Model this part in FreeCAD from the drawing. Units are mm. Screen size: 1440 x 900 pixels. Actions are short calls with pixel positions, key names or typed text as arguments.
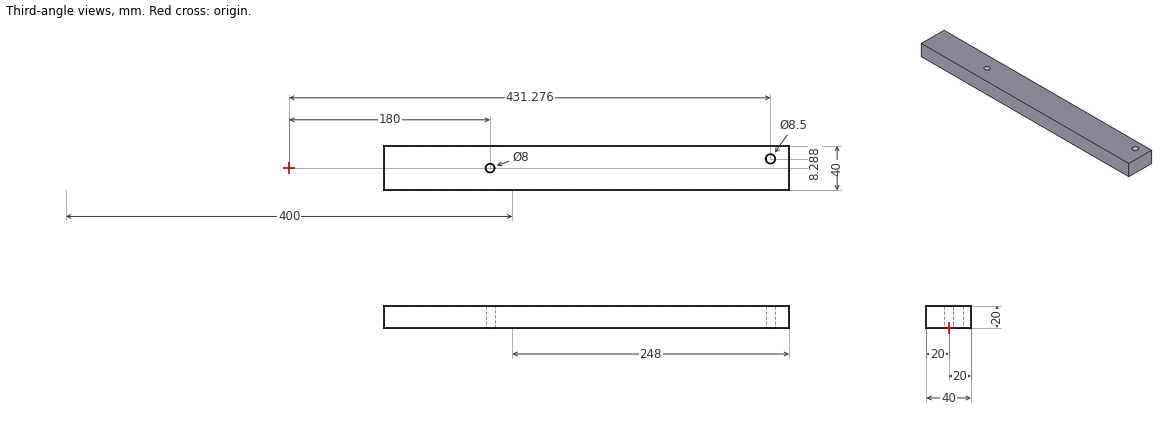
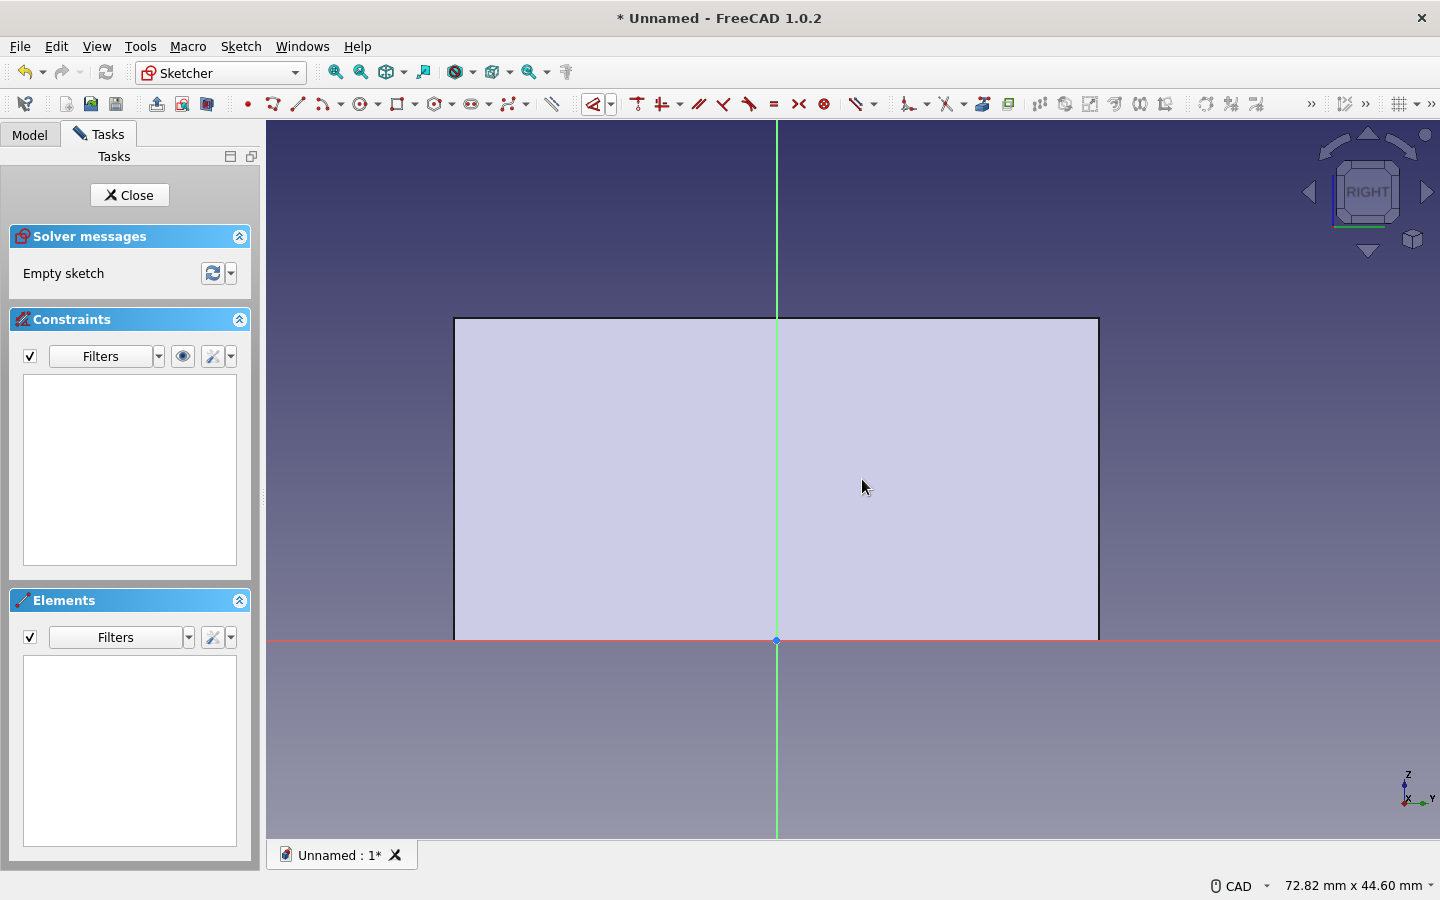
click(396, 104)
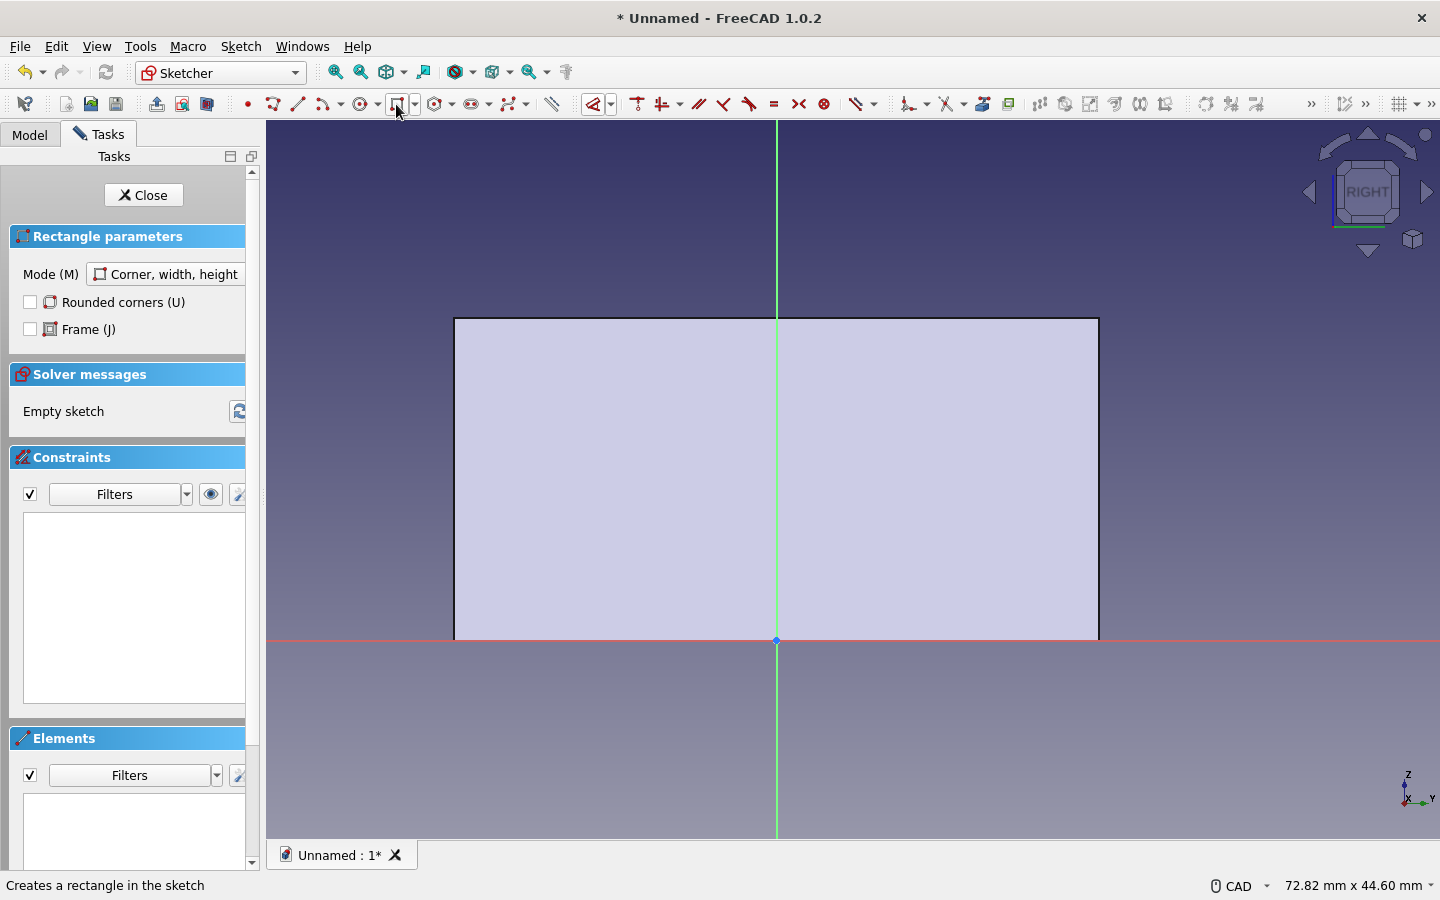
click(454, 318)
click(1099, 641)
key(Escape)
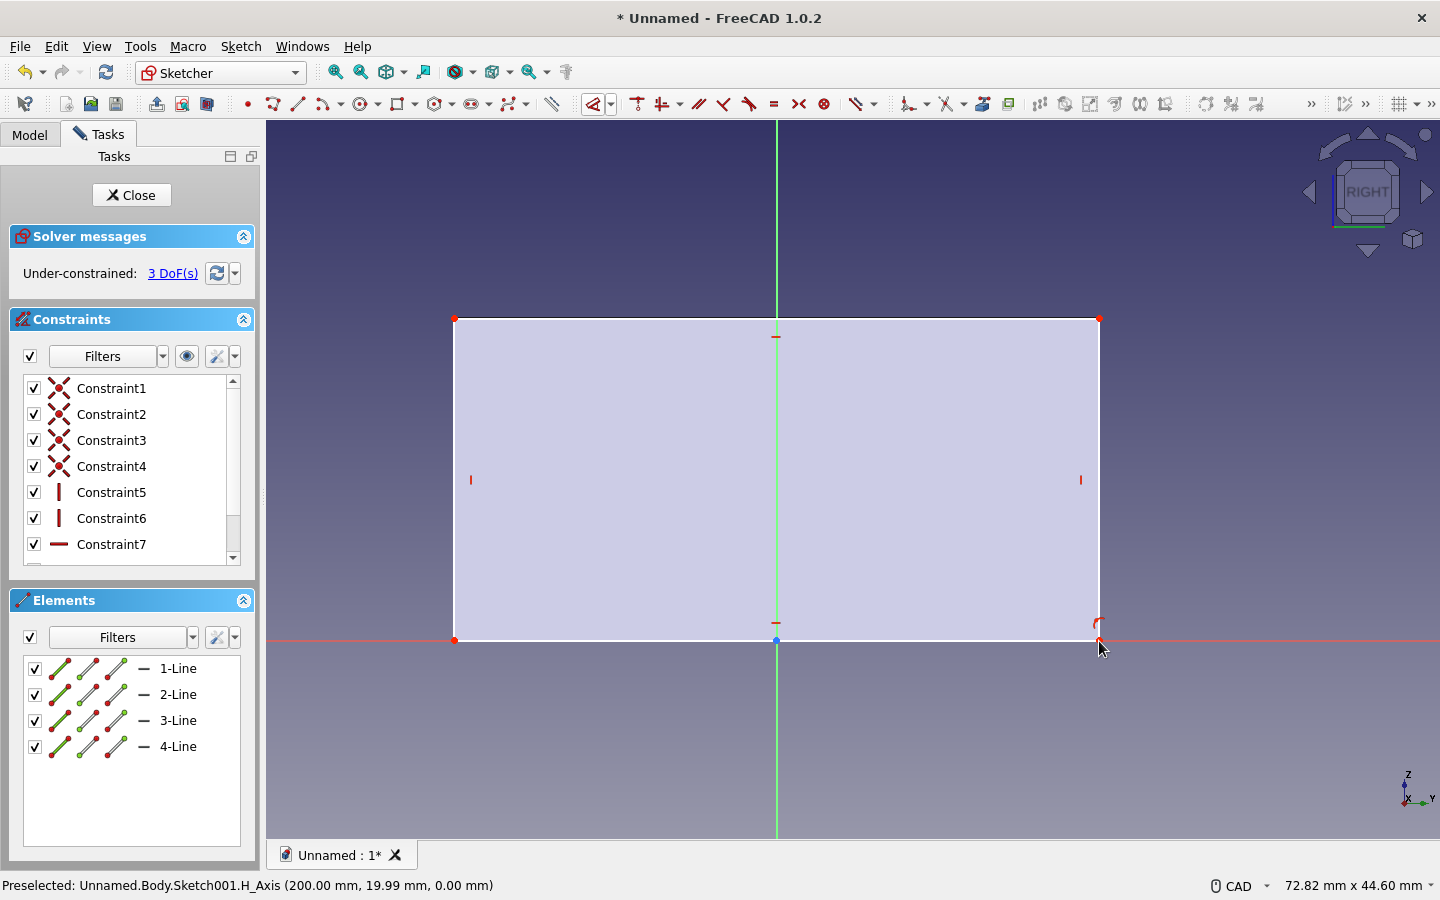
click(454, 416)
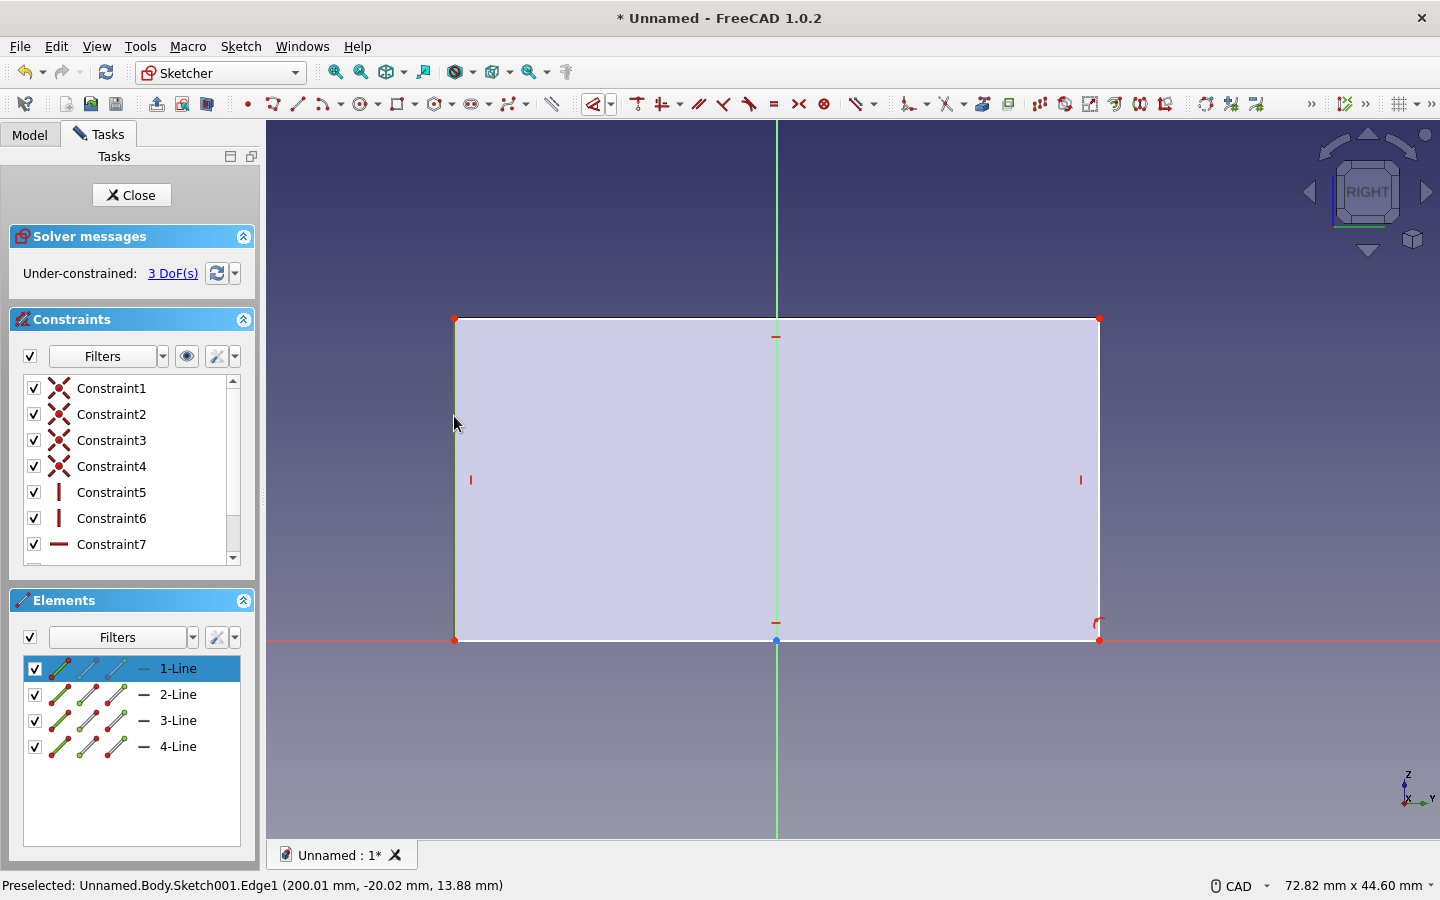
key(i)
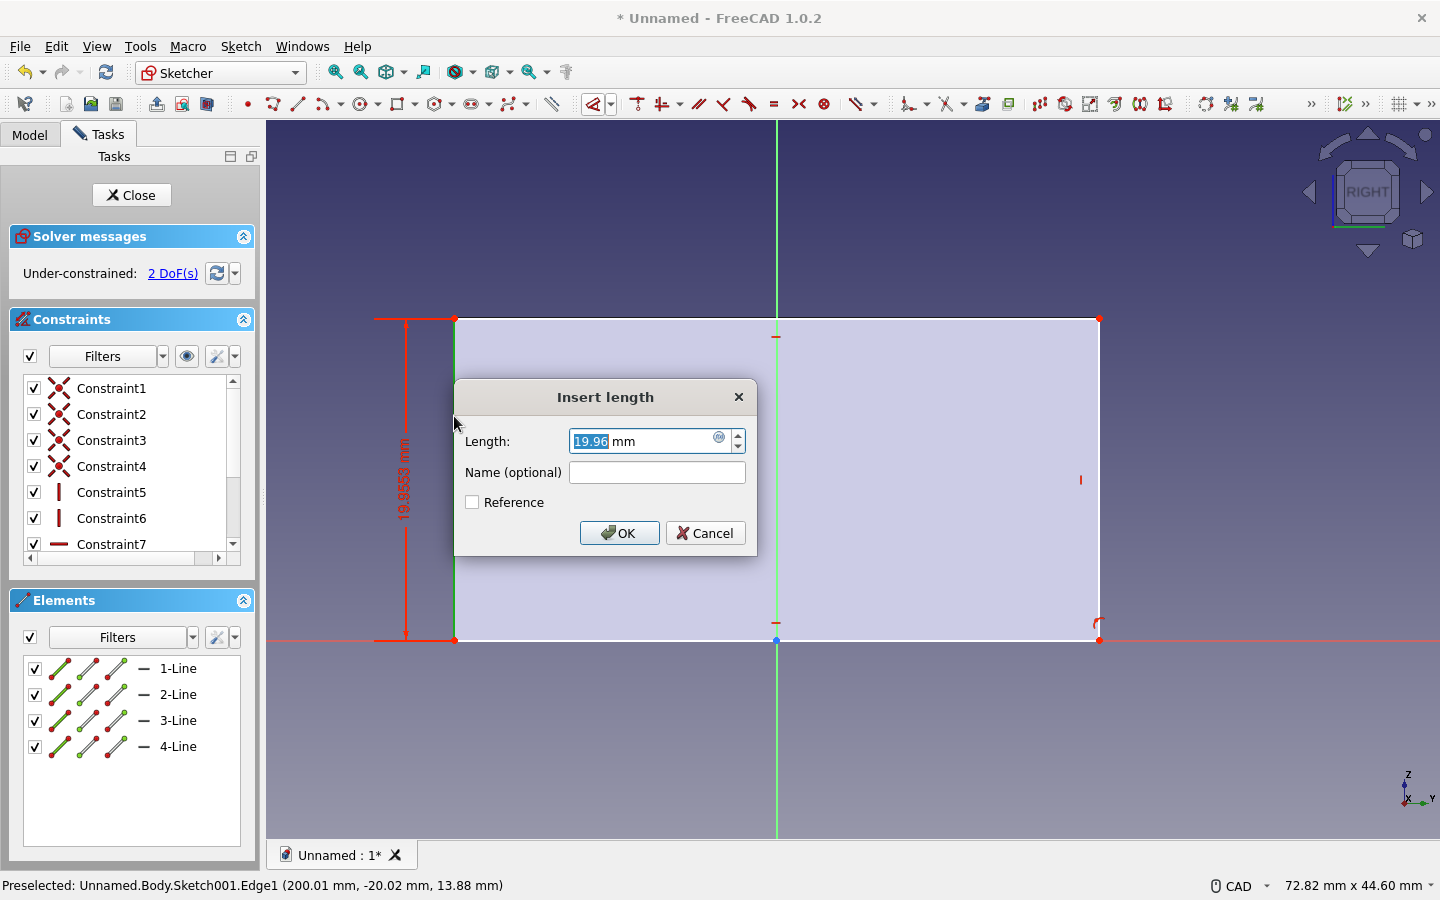
text(20)
key(Return)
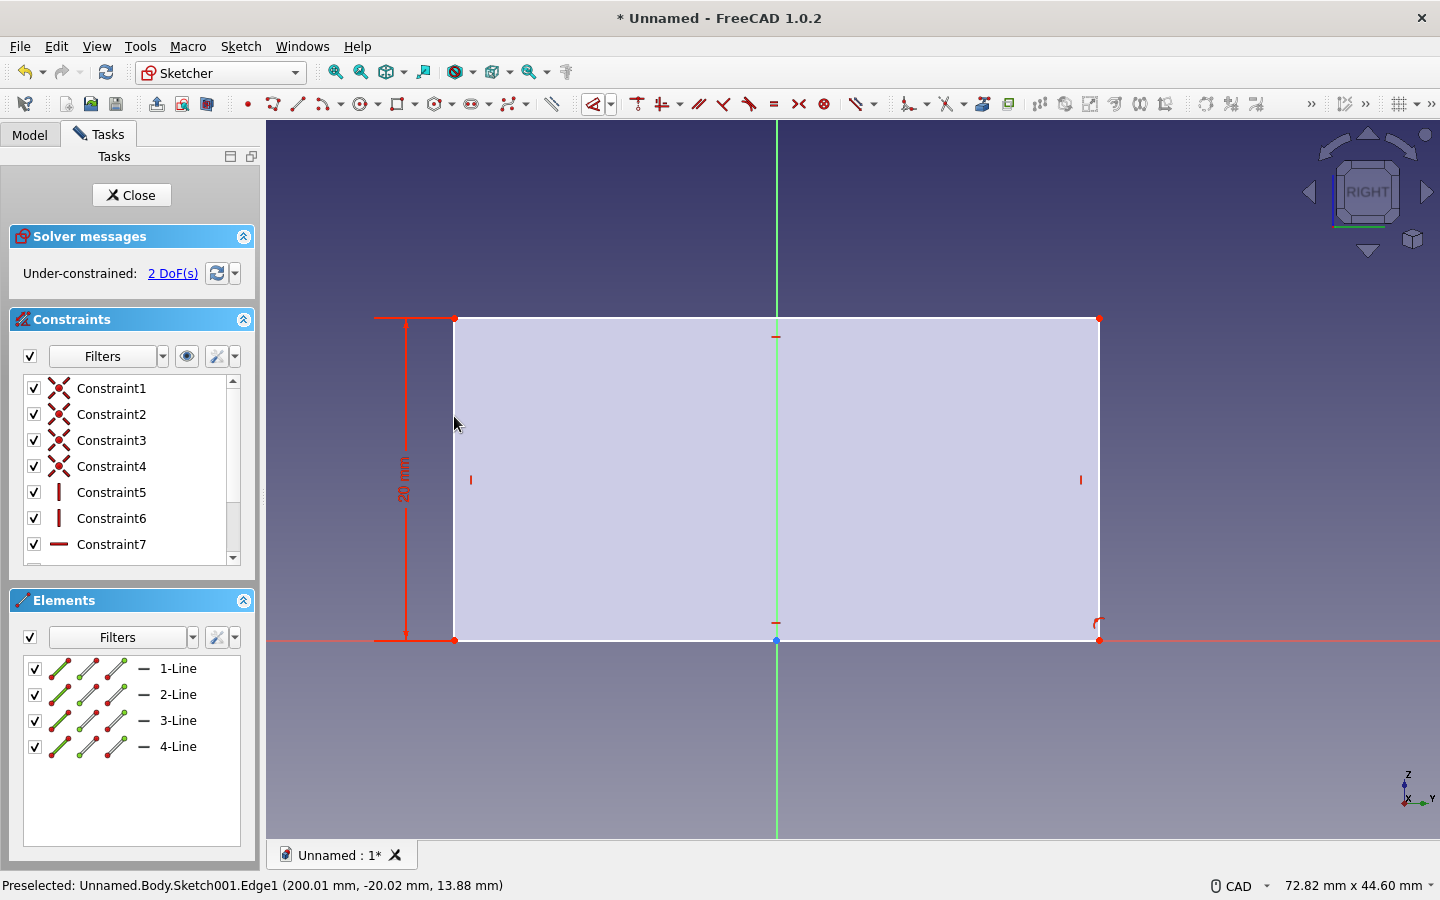
click(647, 641)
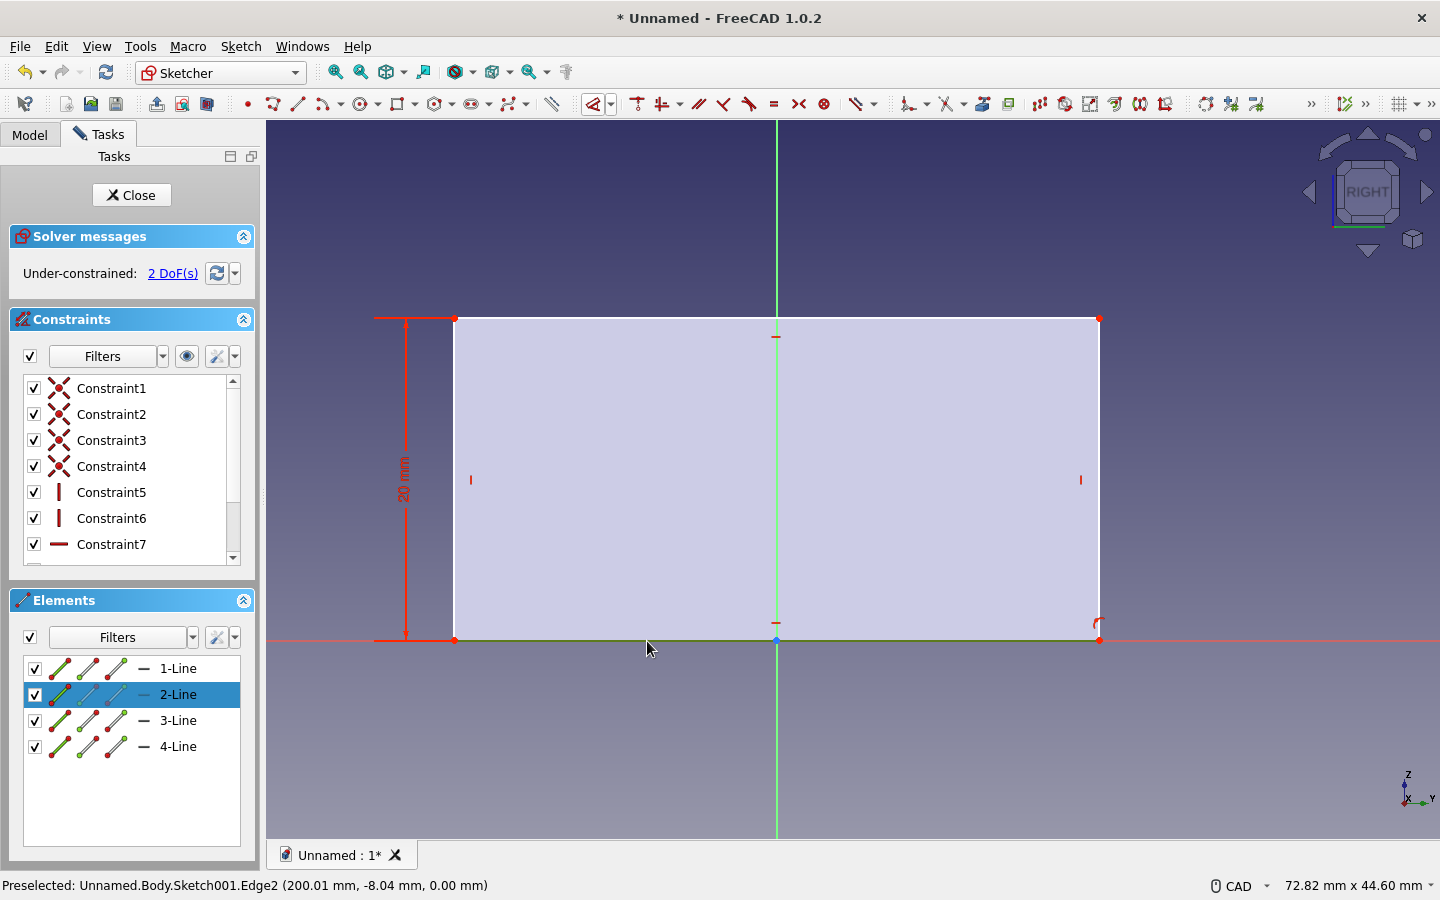
click(610, 104)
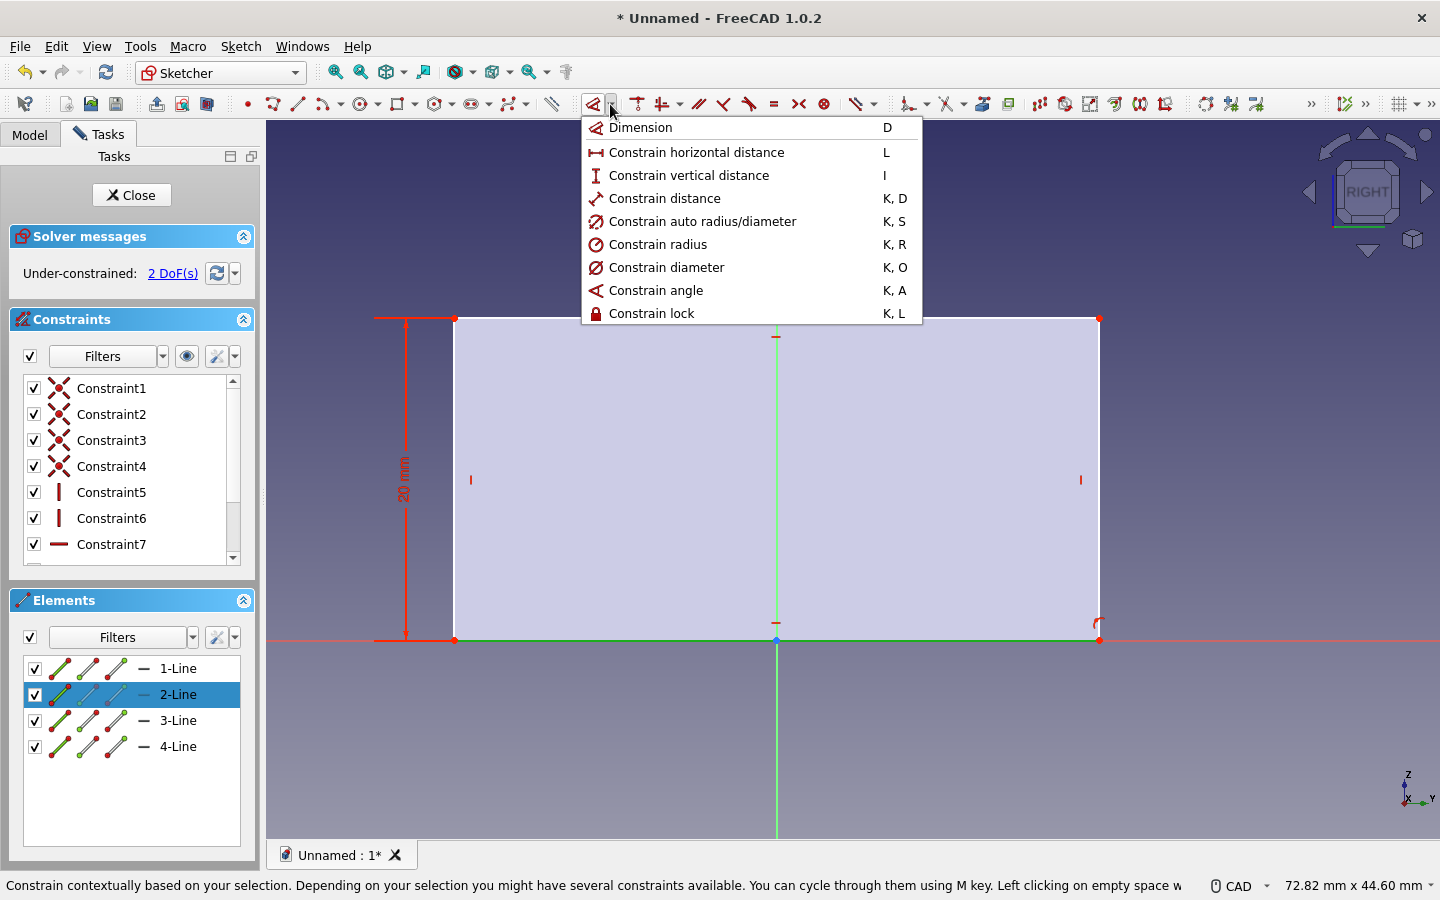
click(752, 152)